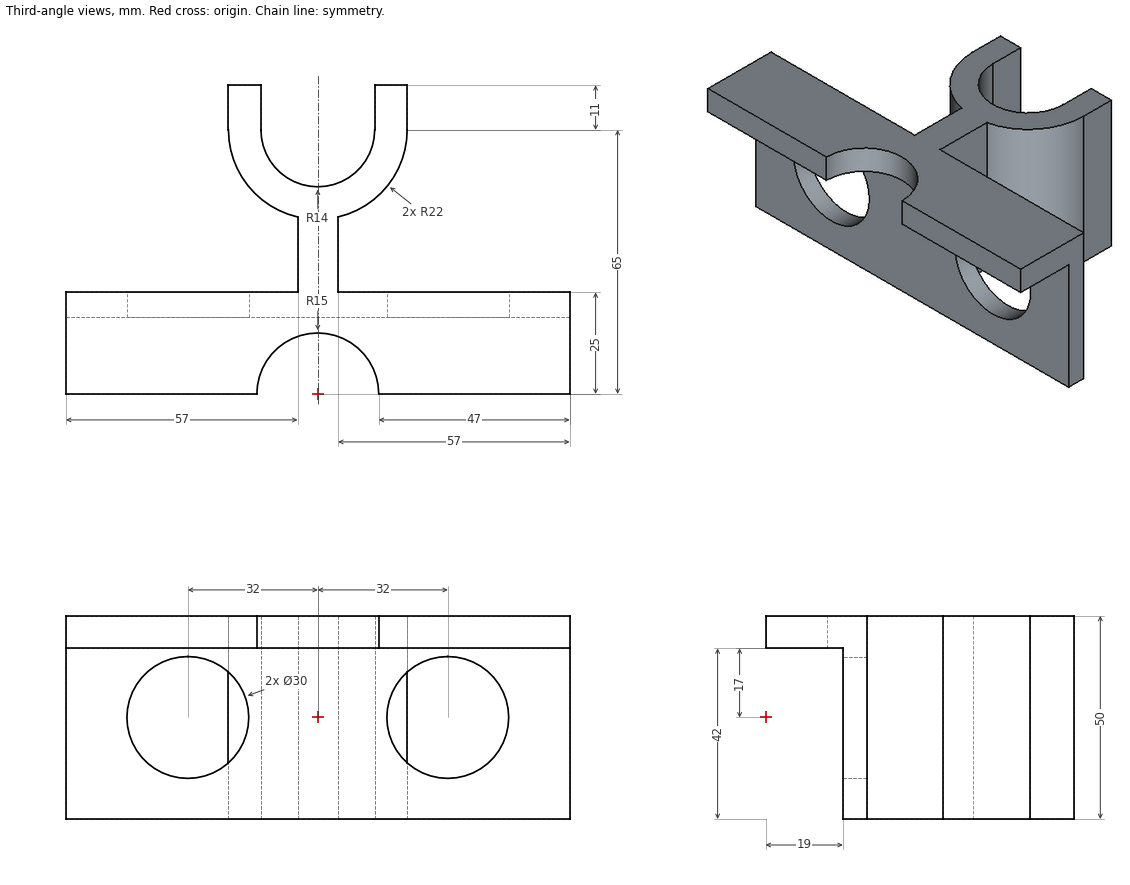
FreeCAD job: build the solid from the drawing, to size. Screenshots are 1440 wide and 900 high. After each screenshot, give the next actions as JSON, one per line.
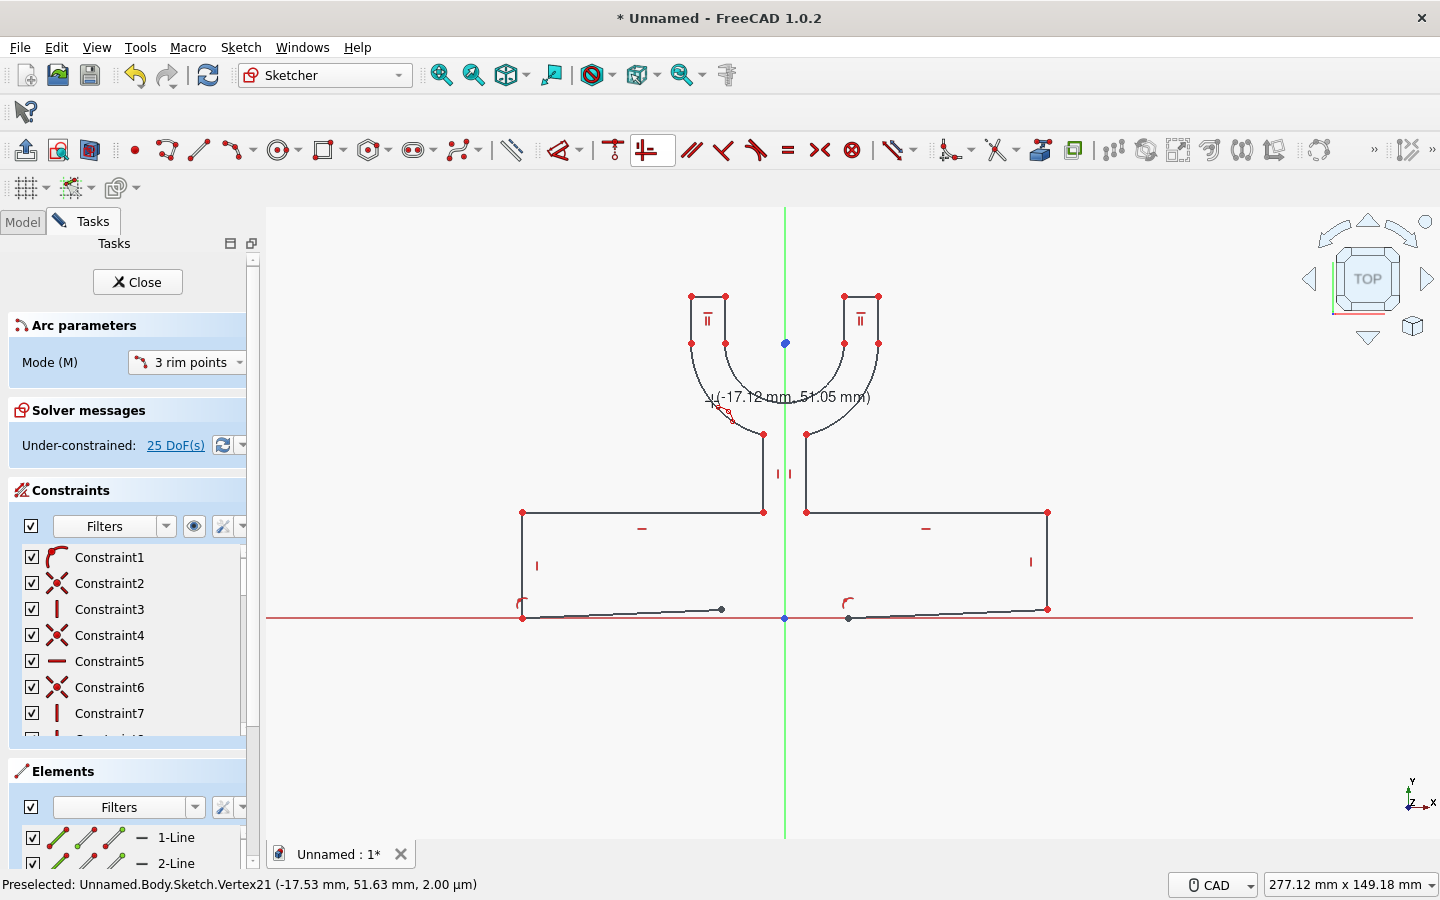
{"action": "left_click", "coordinate": [721, 610]}
{"action": "left_click", "coordinate": [848, 618]}
{"action": "left_click", "coordinate": [804, 558]}
{"action": "key", "text": "Escape"}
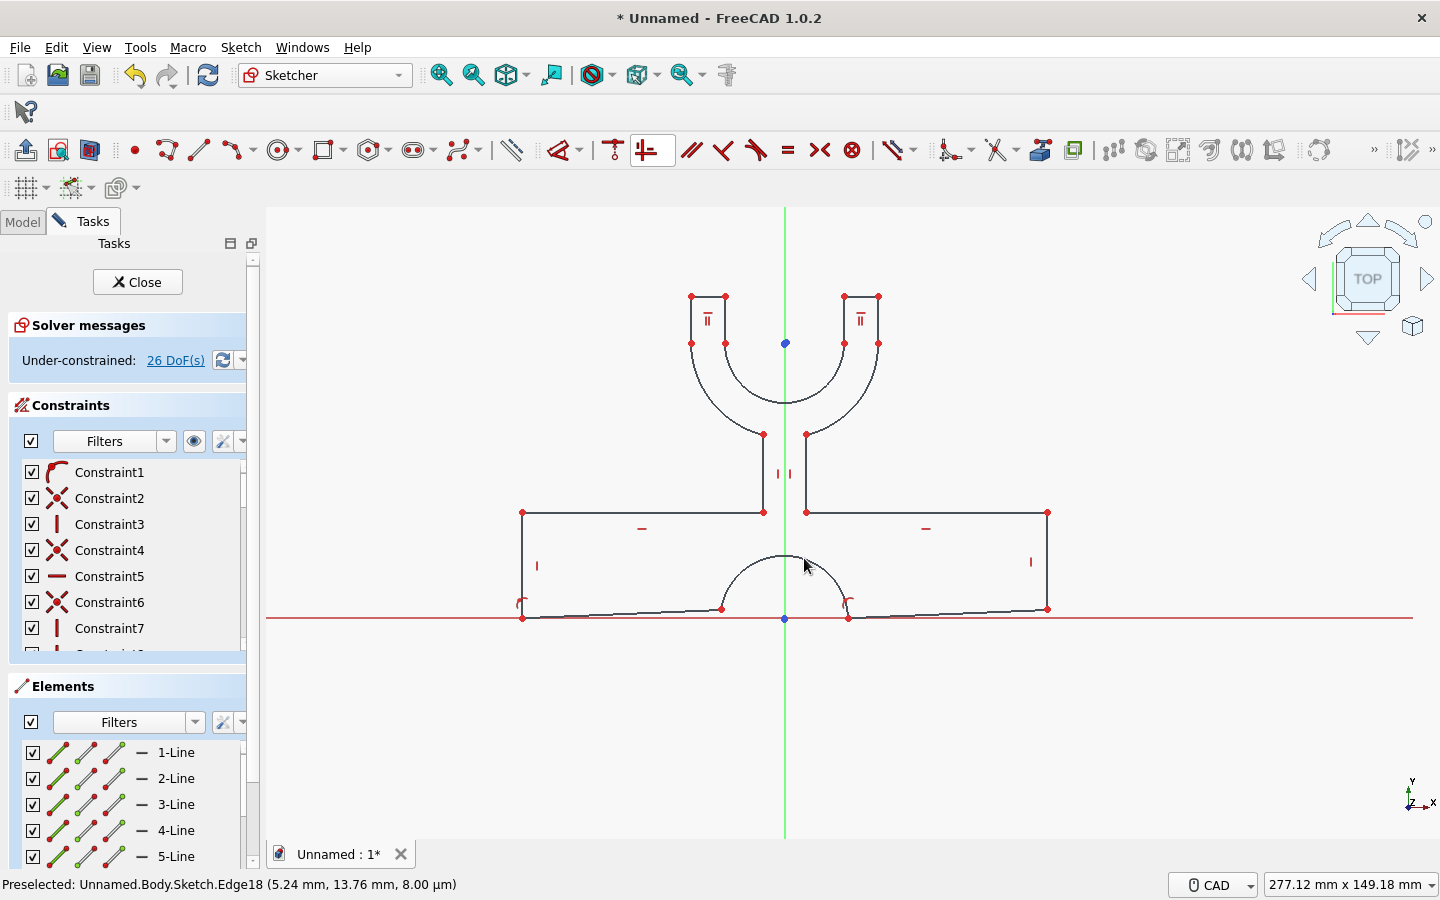
{"action": "left_click", "coordinate": [878, 330]}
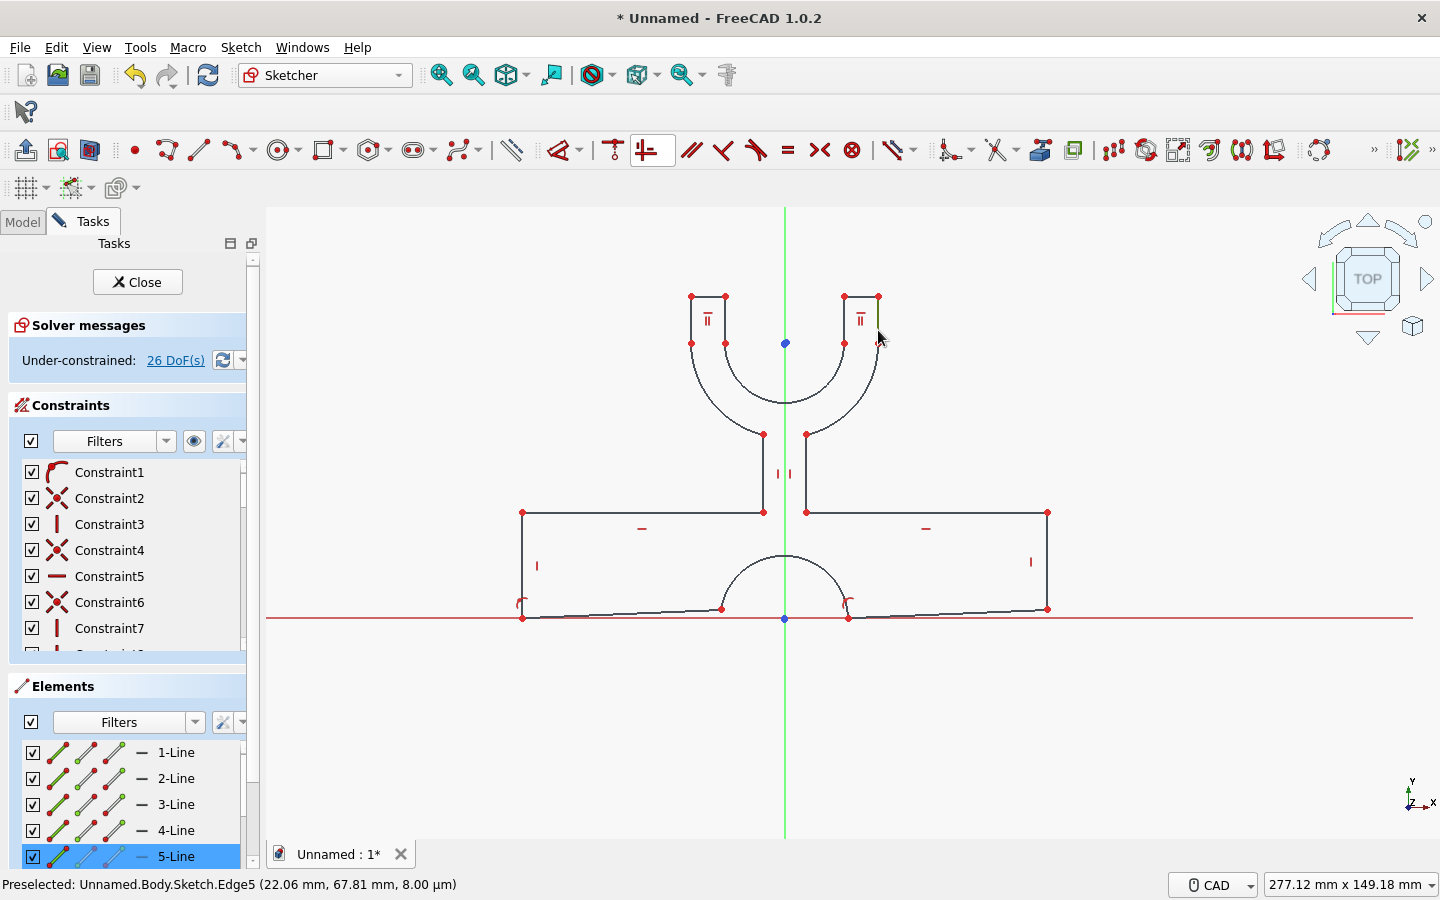
{"action": "left_click", "coordinate": [840, 419]}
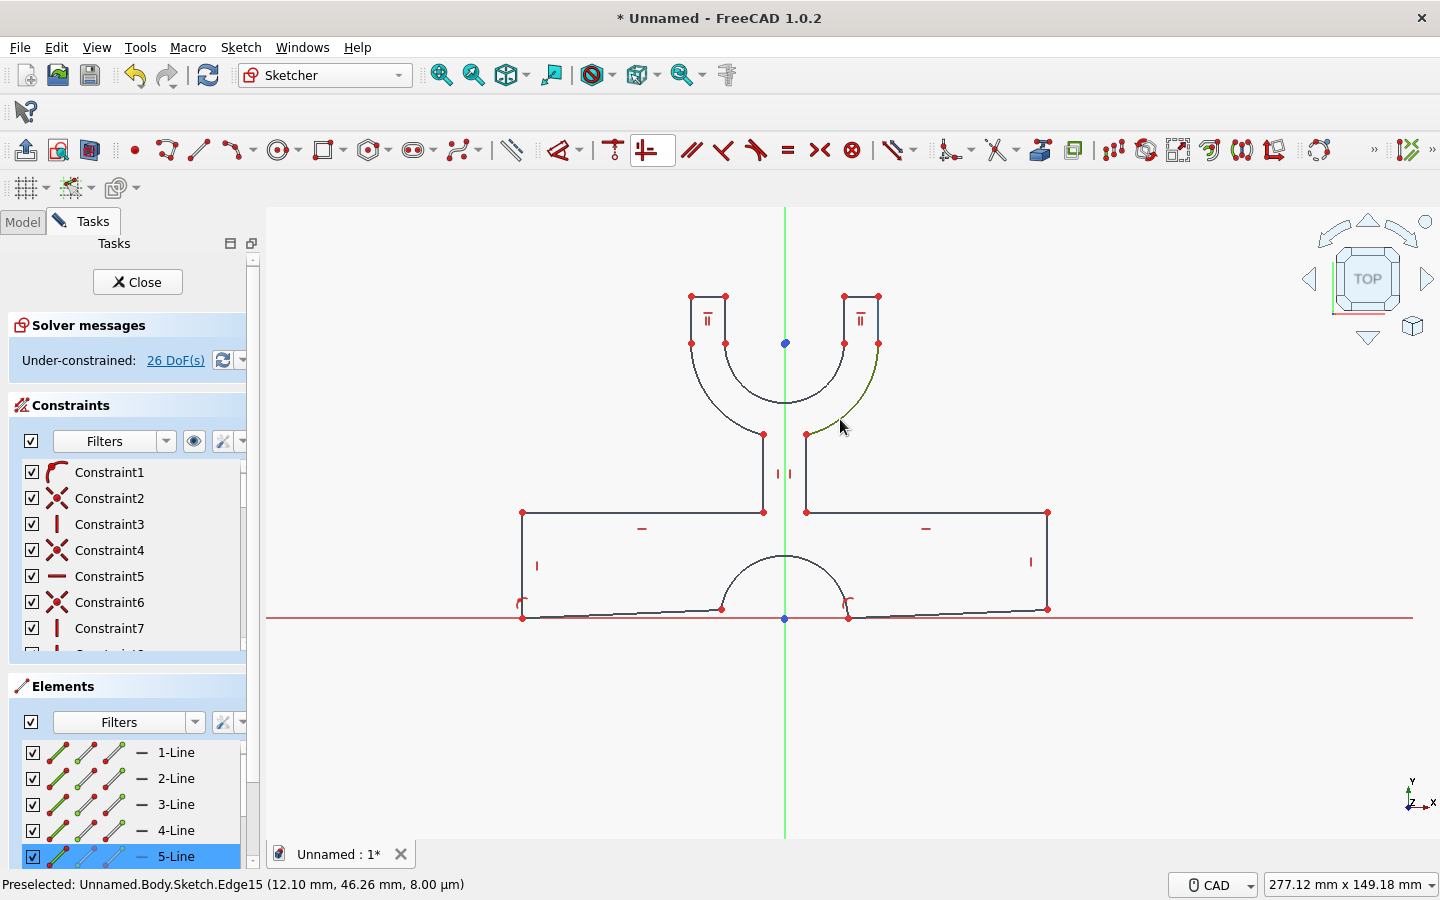
{"action": "left_click", "coordinate": [756, 150]}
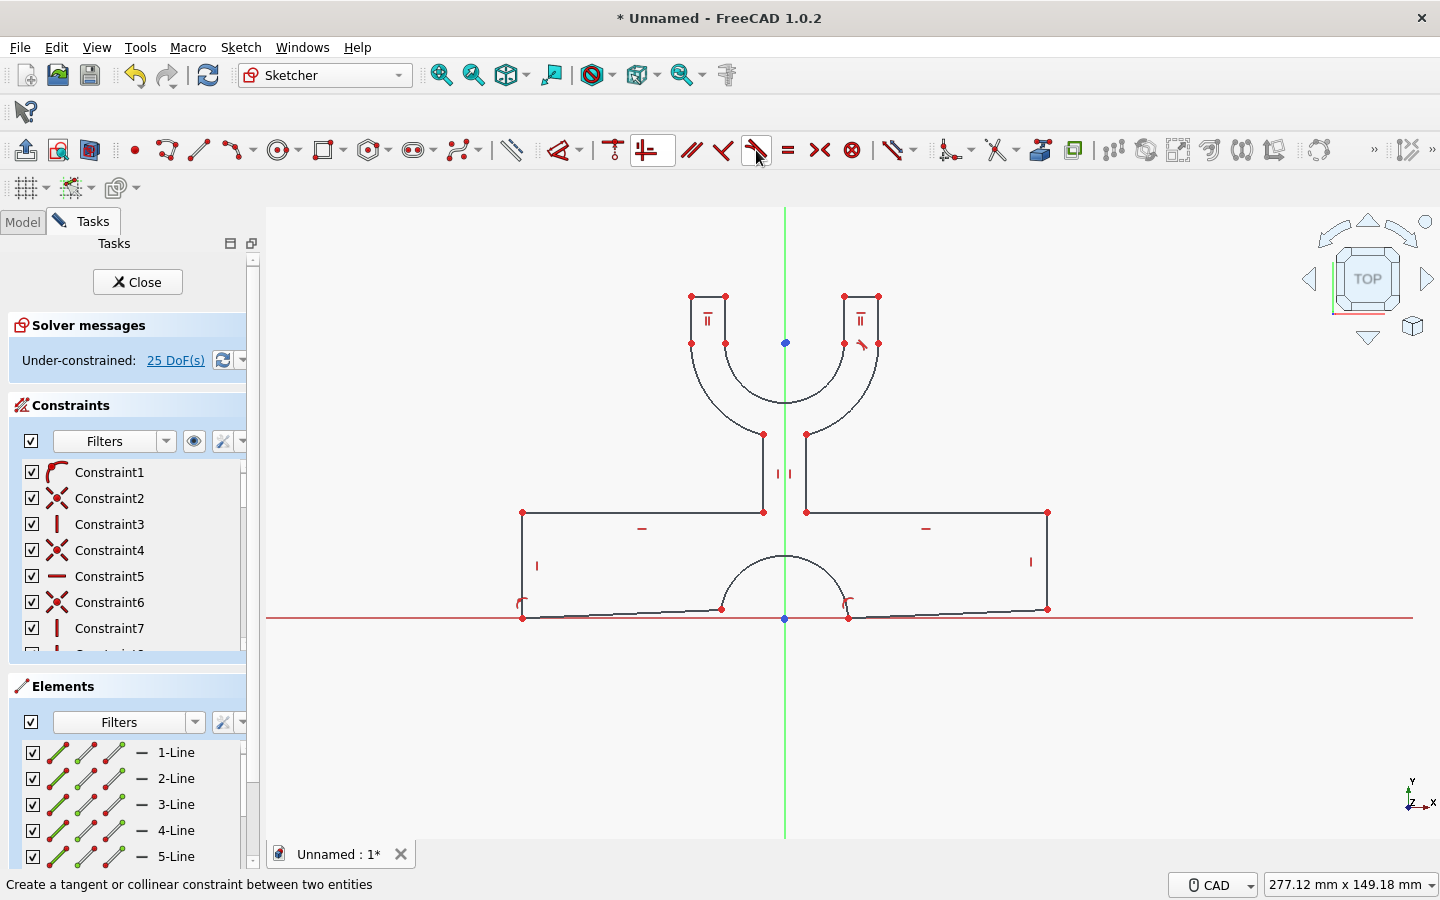
{"action": "left_click", "coordinate": [844, 311]}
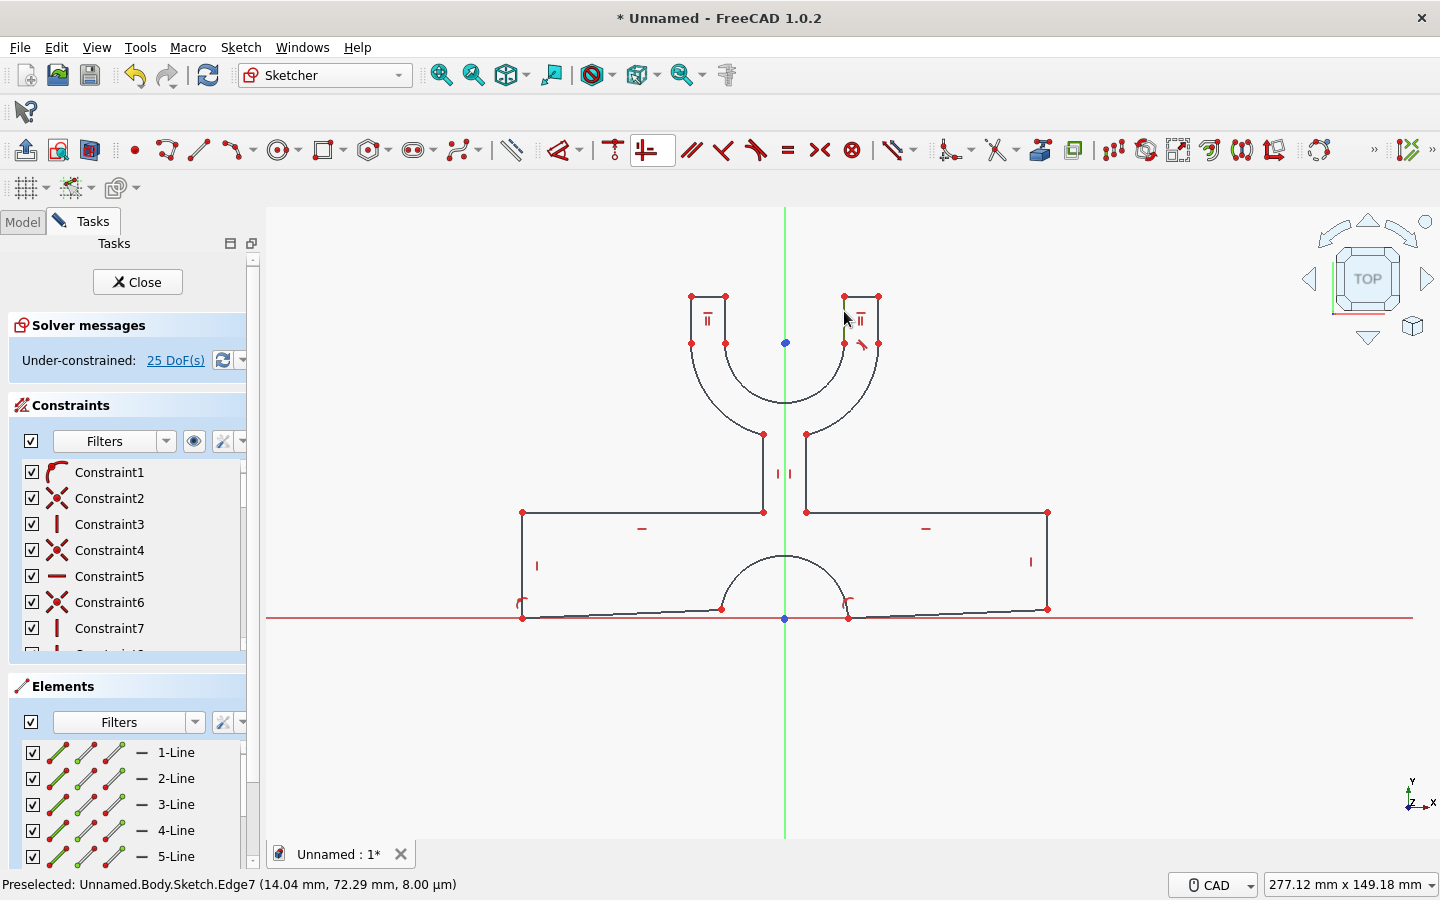
{"action": "left_click", "coordinate": [750, 392]}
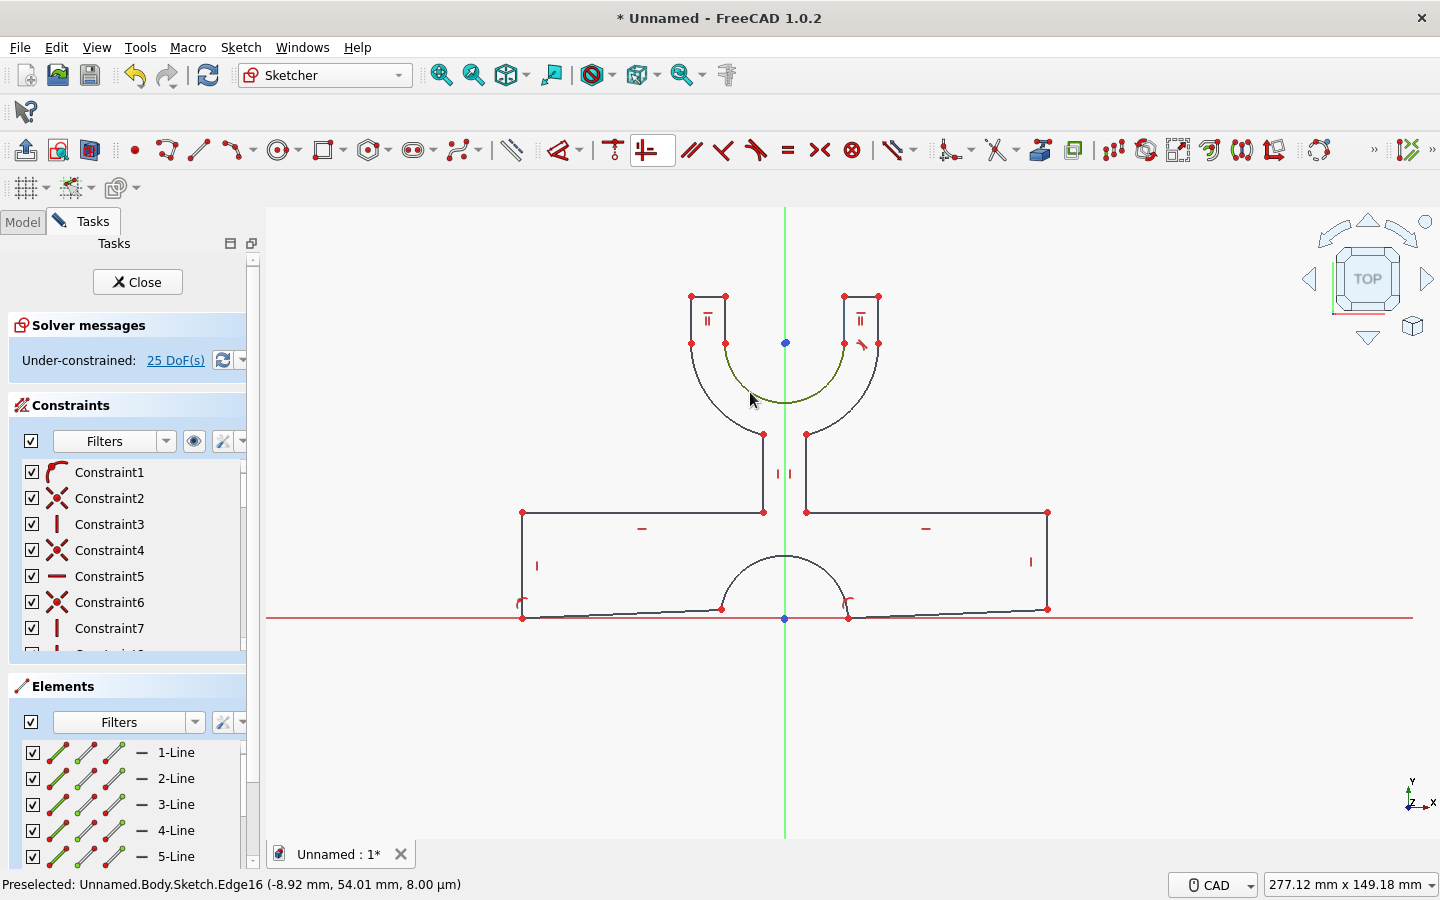
{"action": "left_click", "coordinate": [756, 150]}